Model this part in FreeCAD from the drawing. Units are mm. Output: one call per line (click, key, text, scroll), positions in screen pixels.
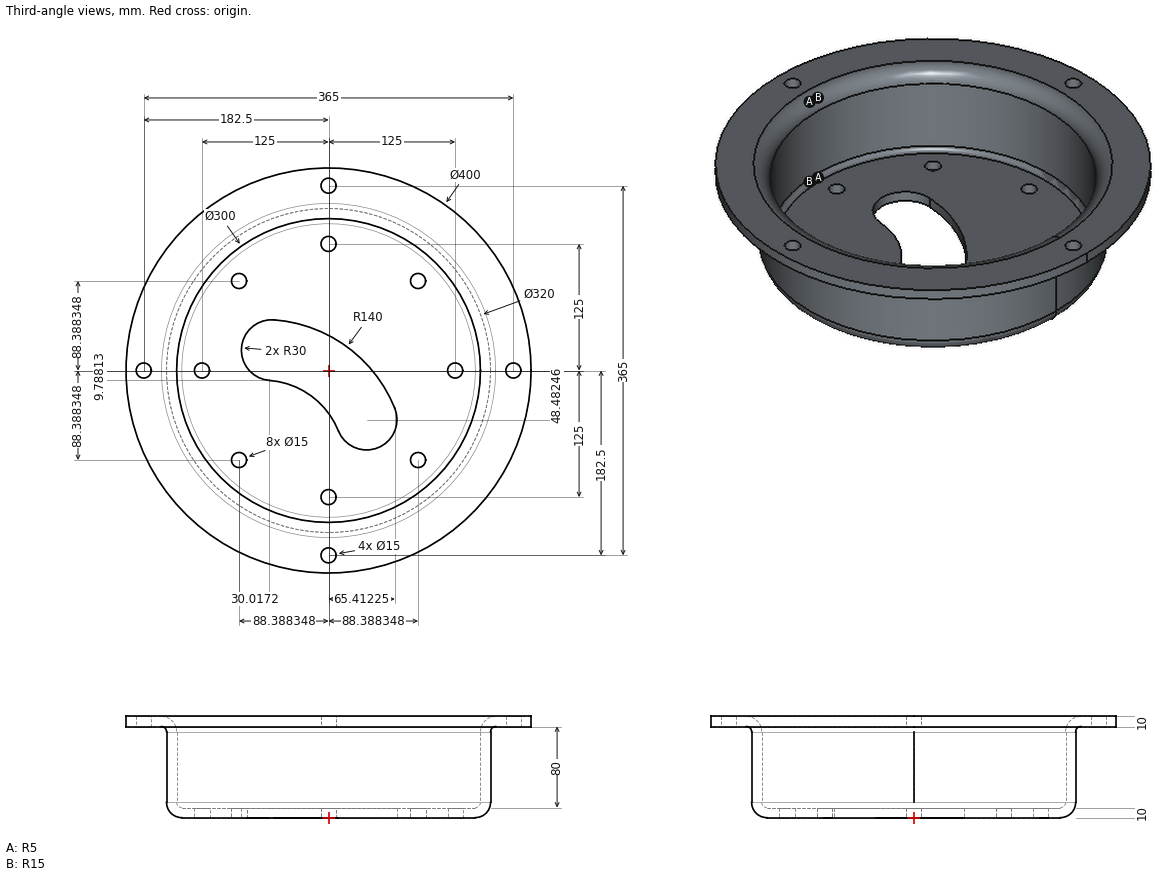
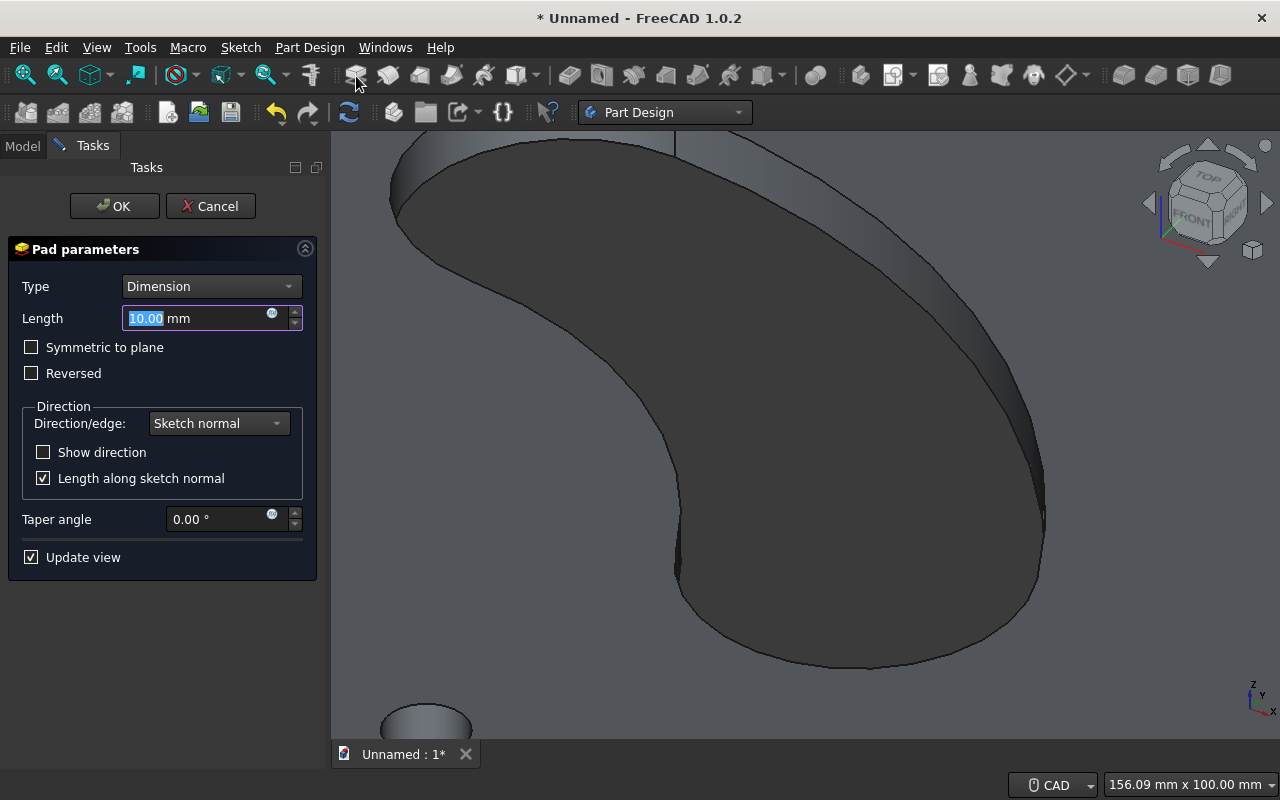
text(10)
key(Tab)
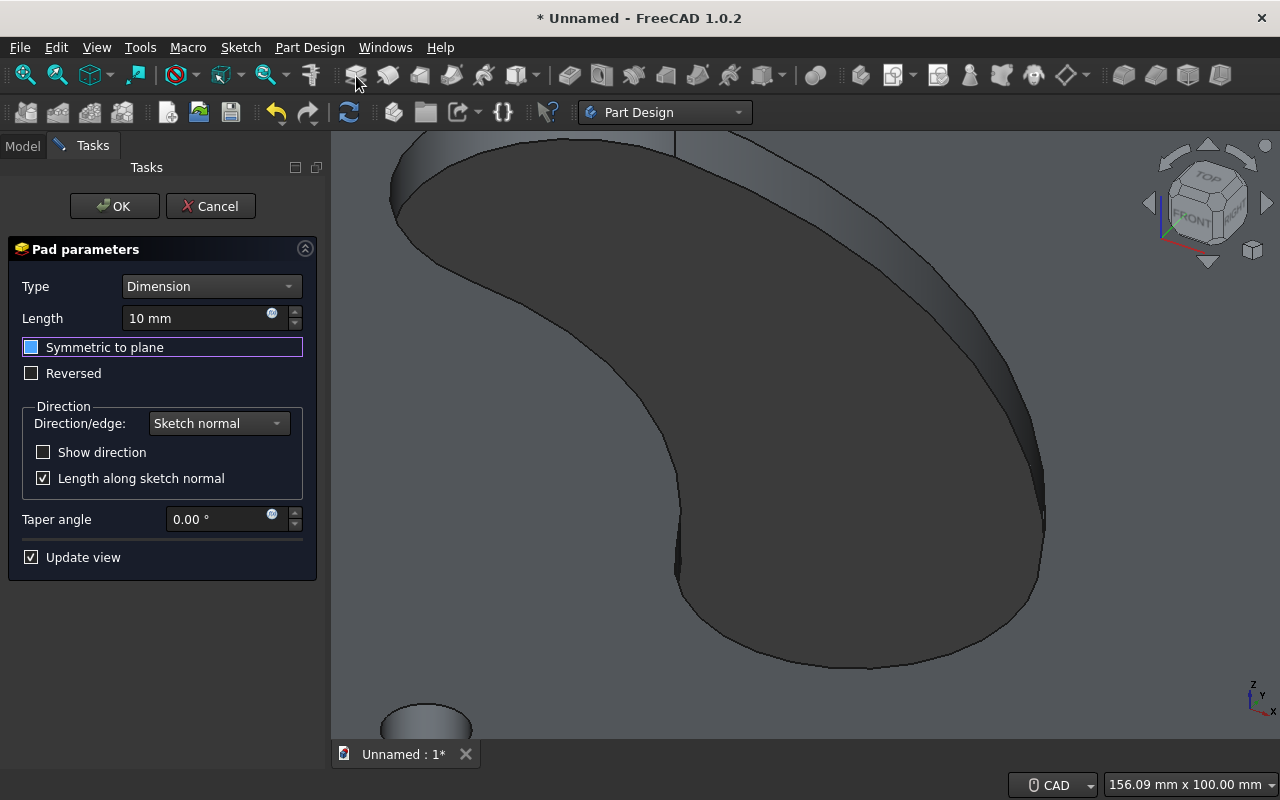
click(115, 206)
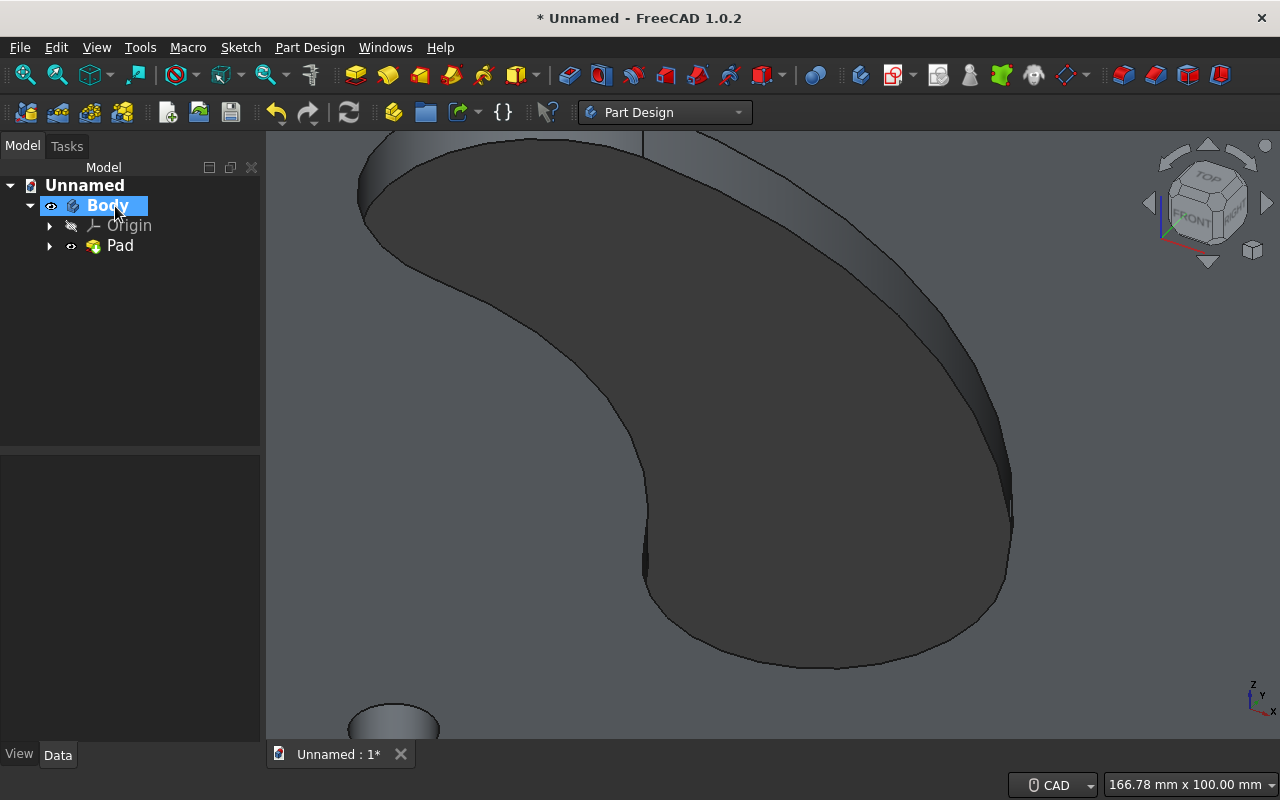
click(26, 76)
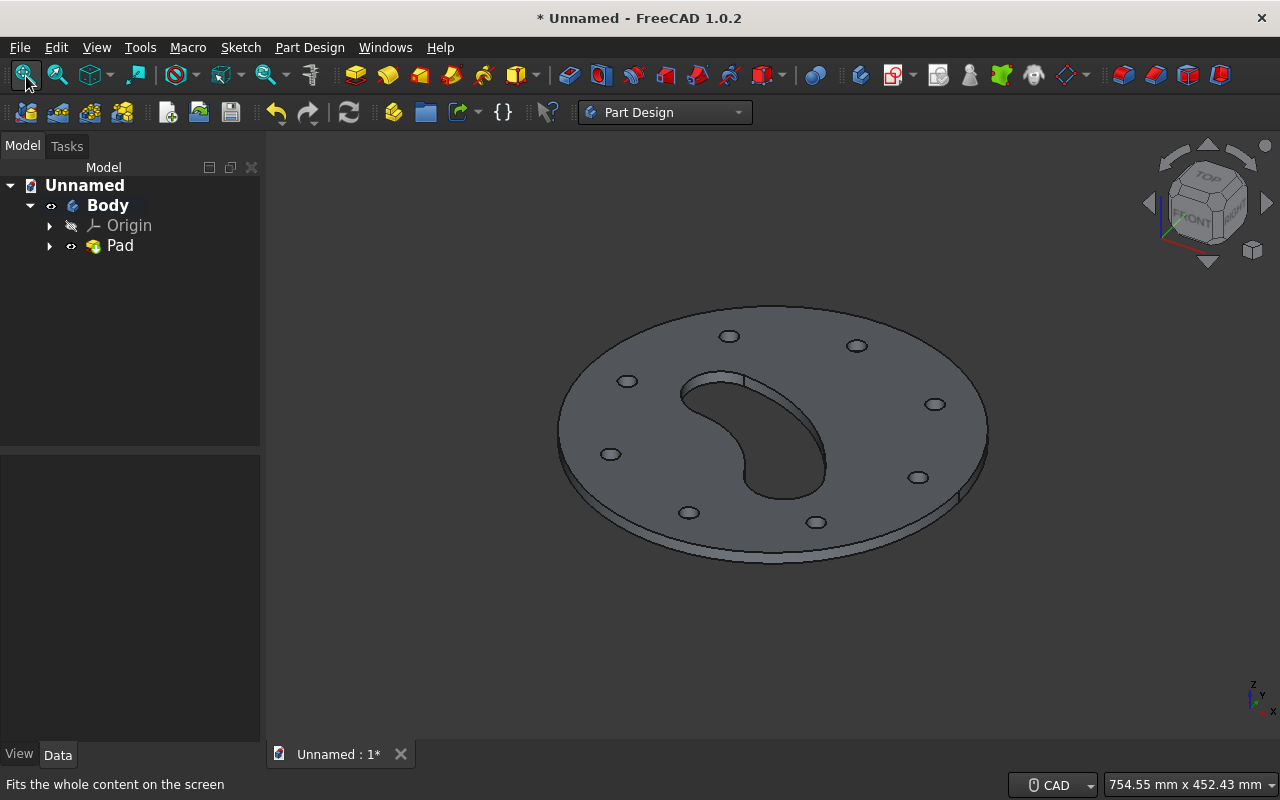
click(781, 350)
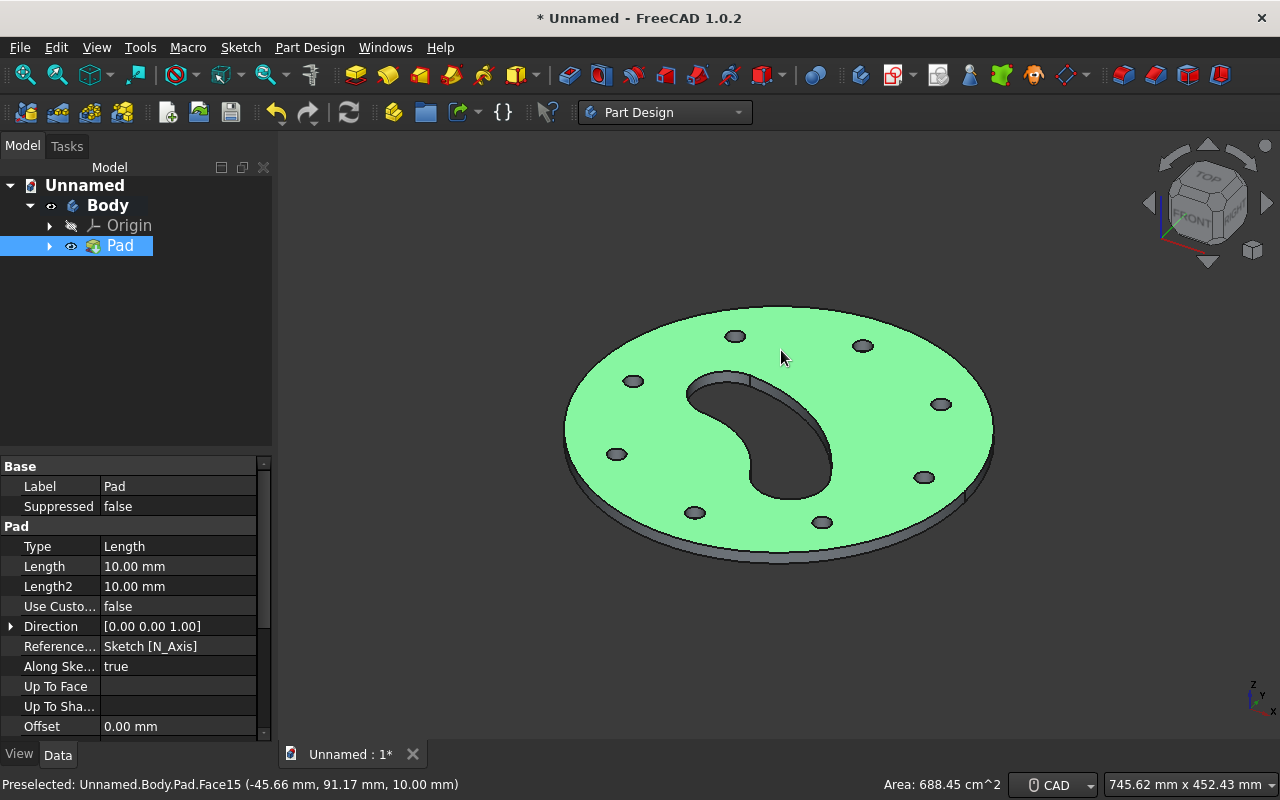
click(894, 76)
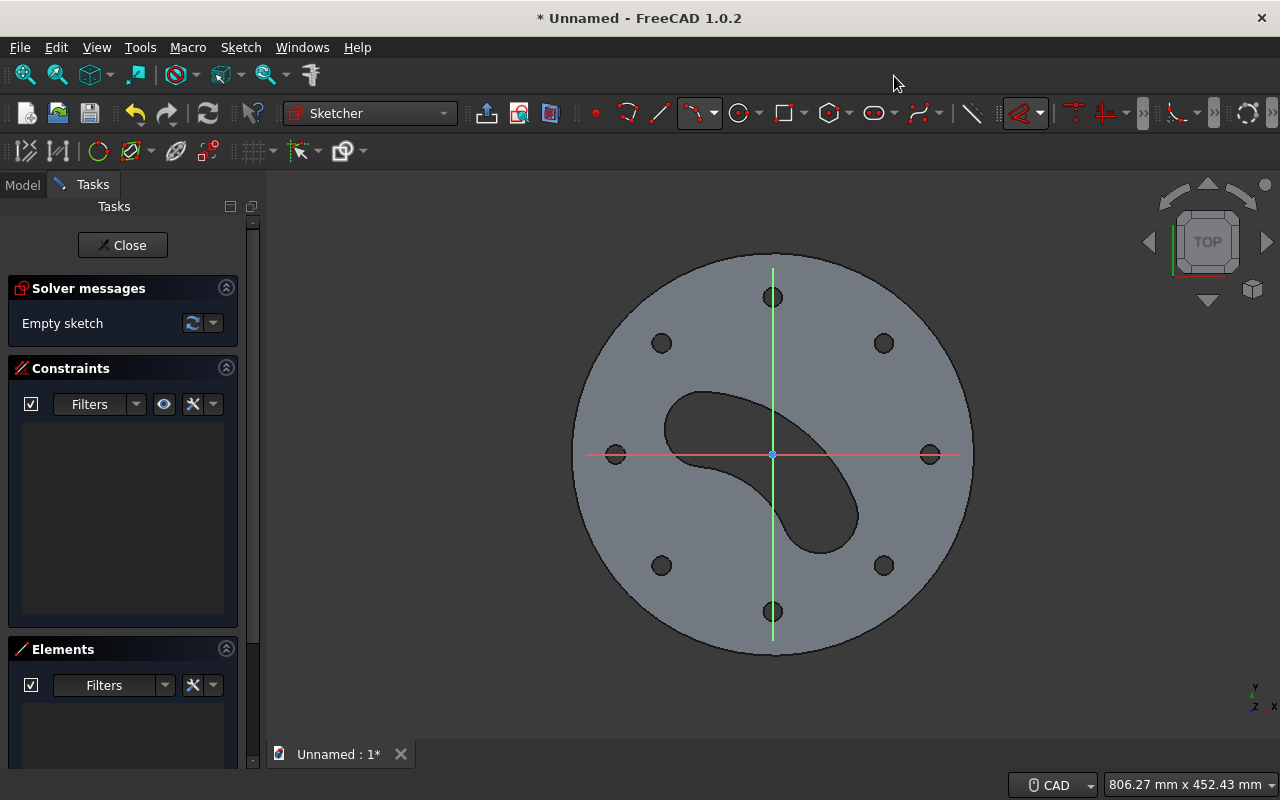
click(740, 114)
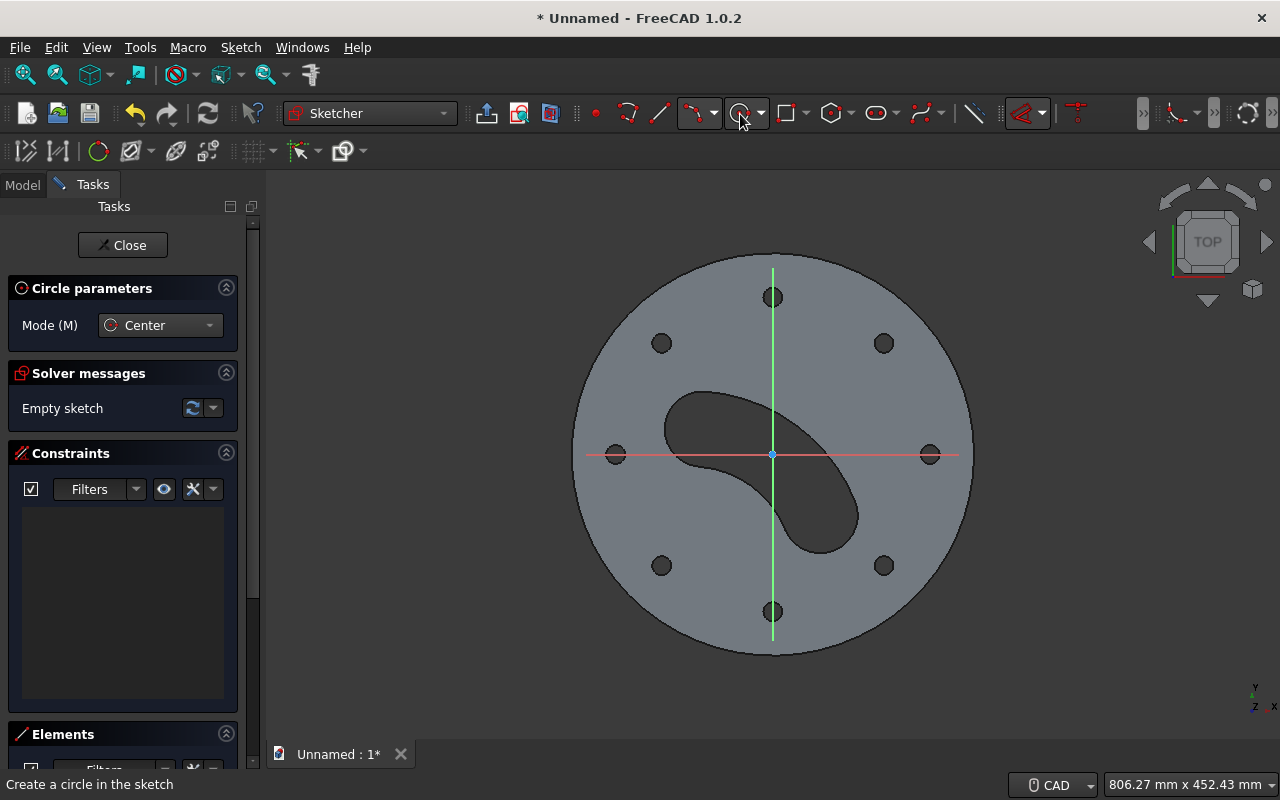
click(773, 454)
click(915, 312)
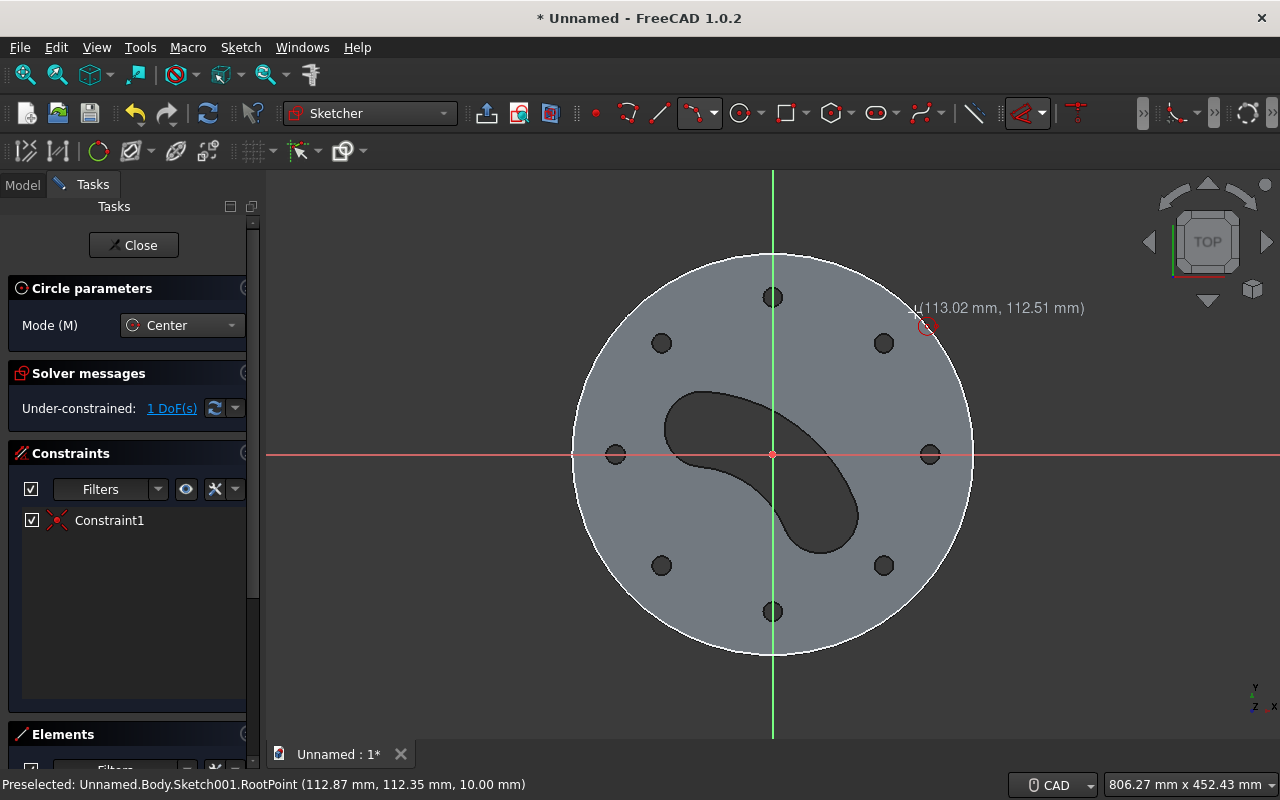
click(773, 454)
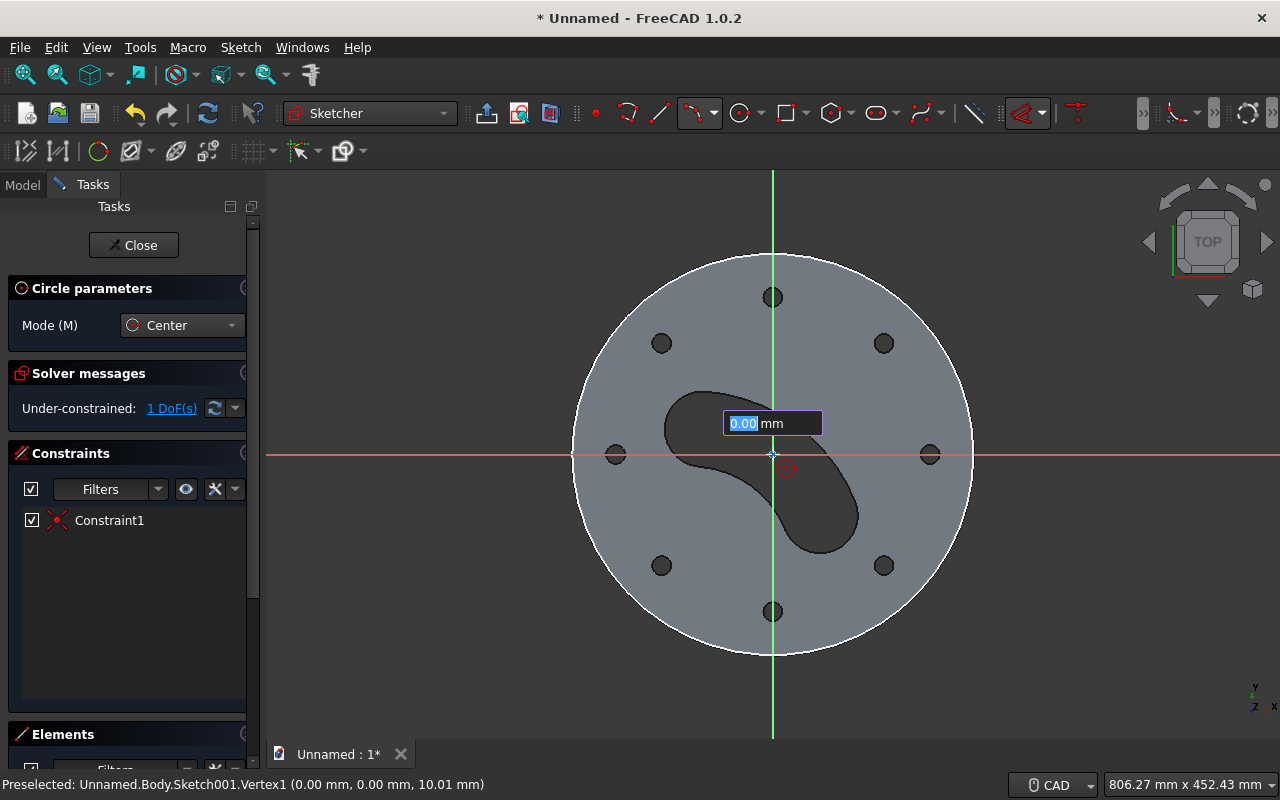
scroll(906, 321, up, 2)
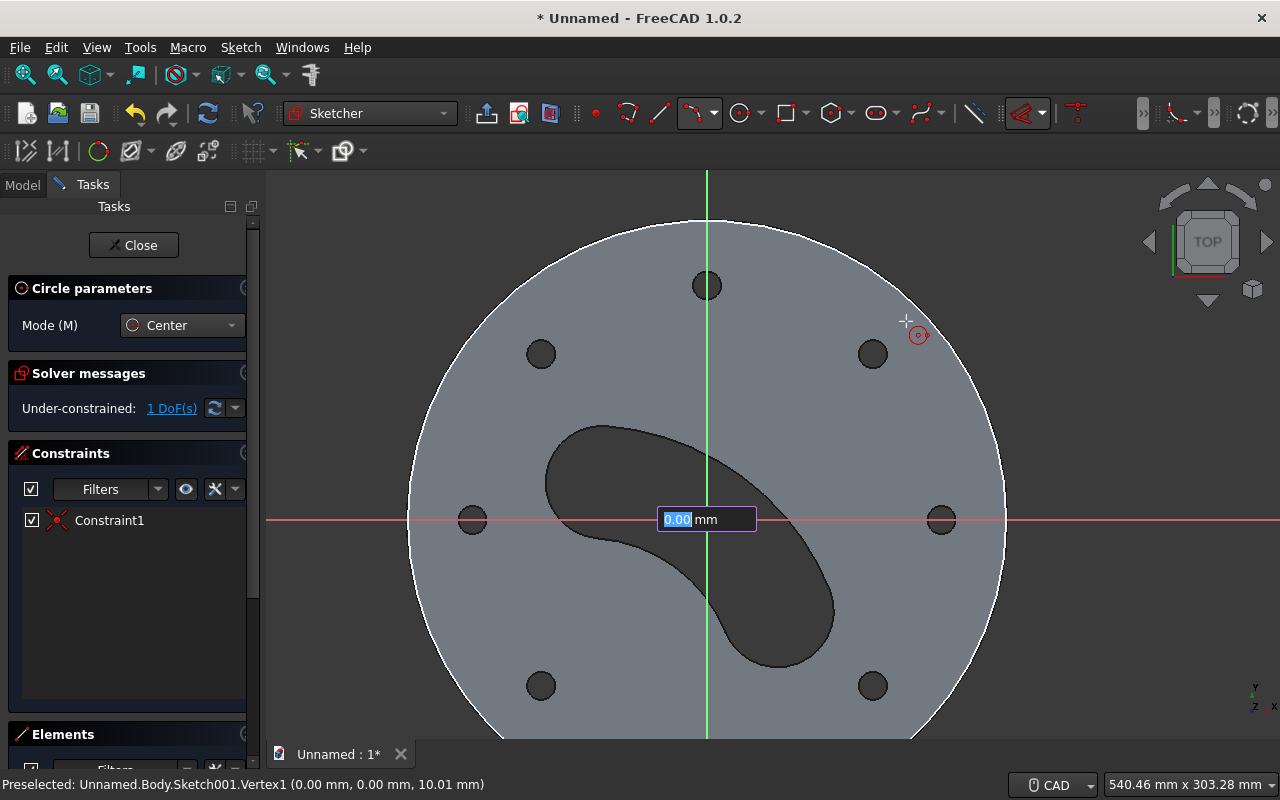
click(906, 321)
key(Escape)